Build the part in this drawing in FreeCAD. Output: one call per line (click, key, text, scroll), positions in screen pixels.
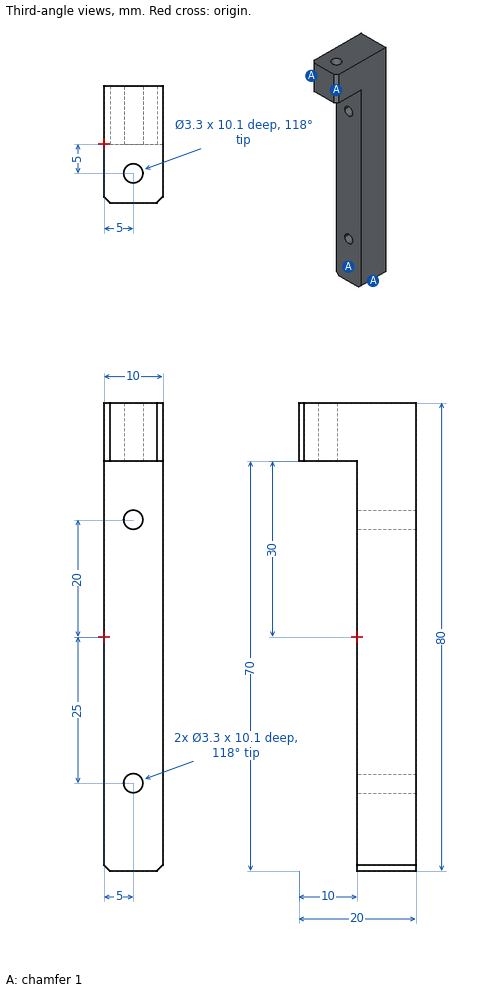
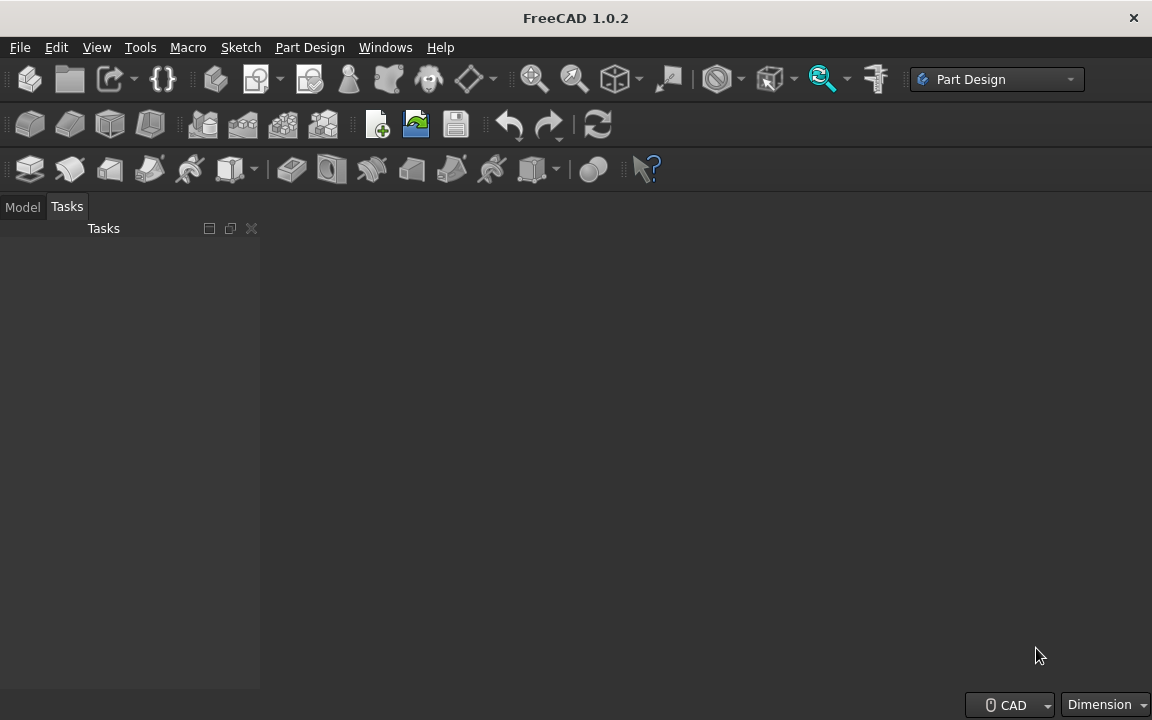
key(ctrl+n)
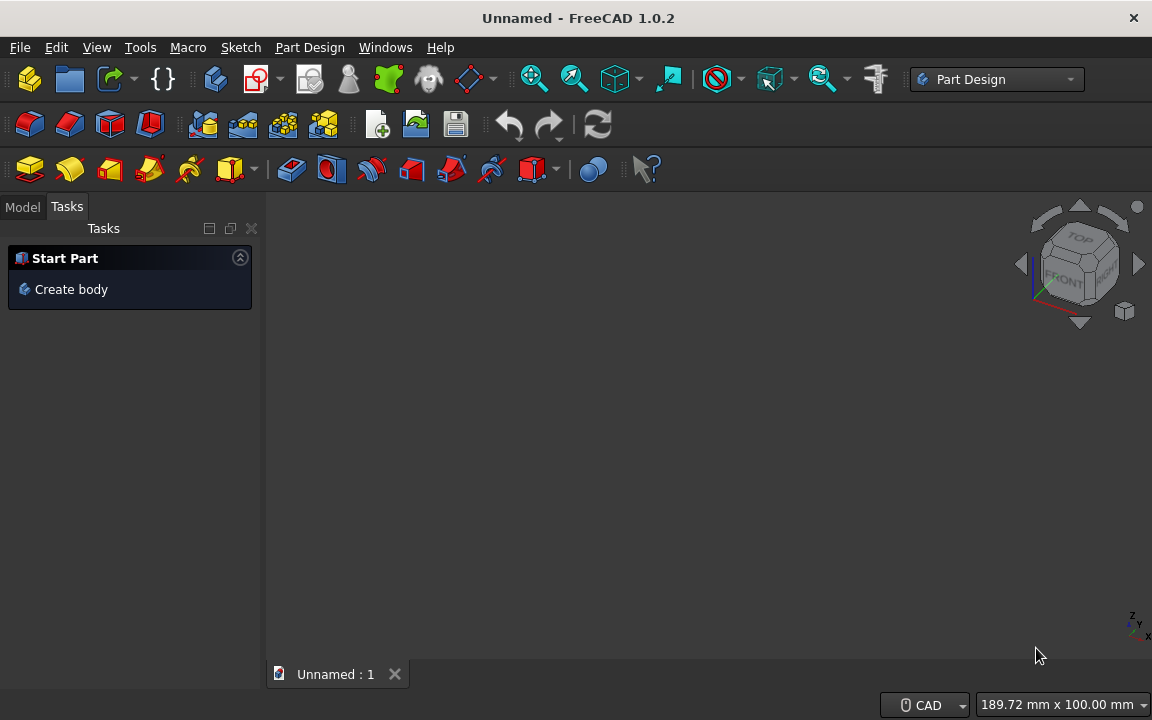
click(256, 80)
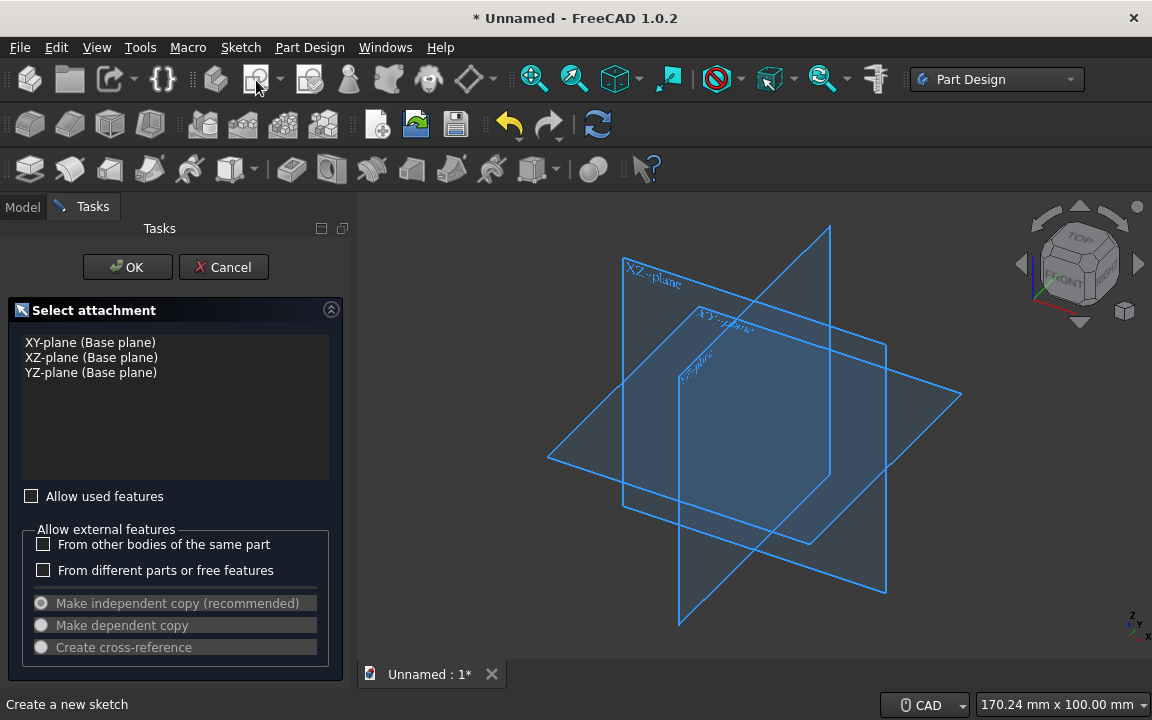
click(82, 372)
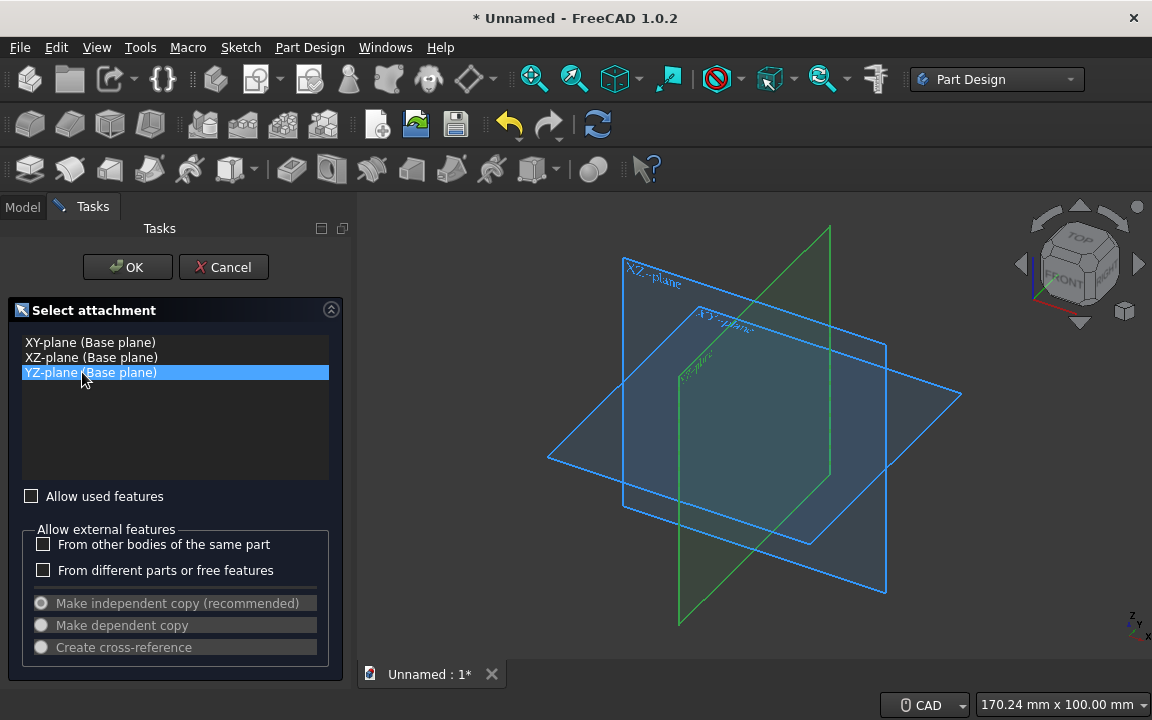
click(128, 267)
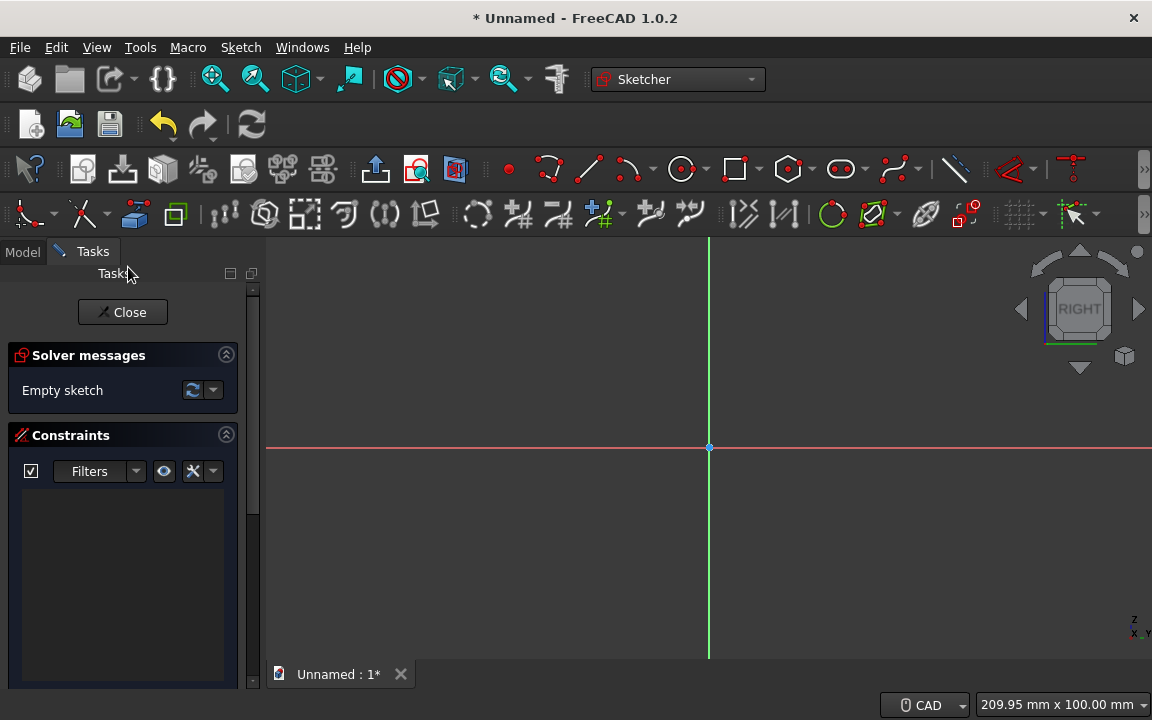
scroll(331, 448, down, 1)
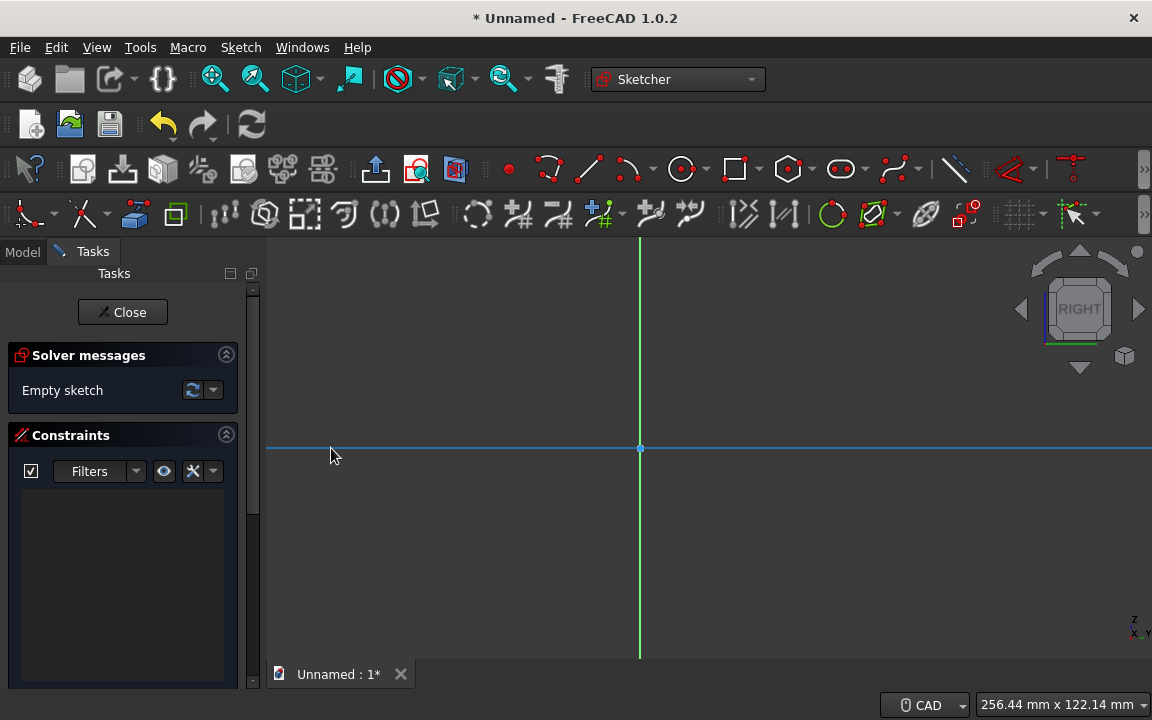
key(g)
key(v)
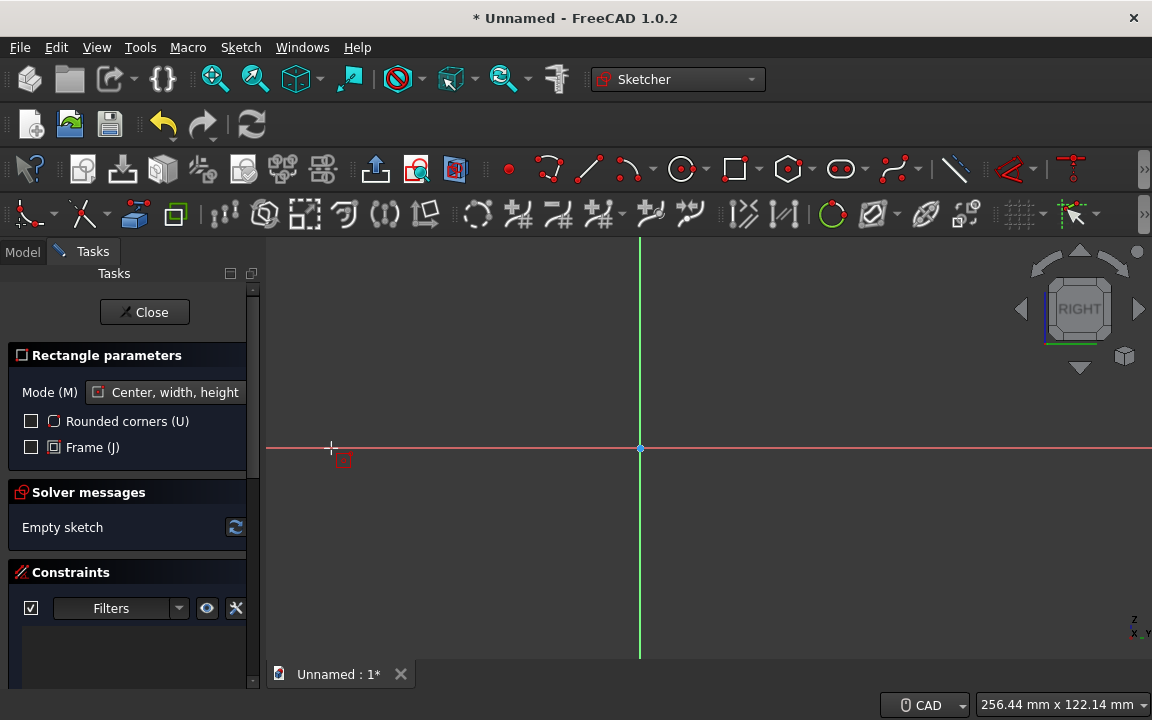
click(640, 448)
move(675, 310)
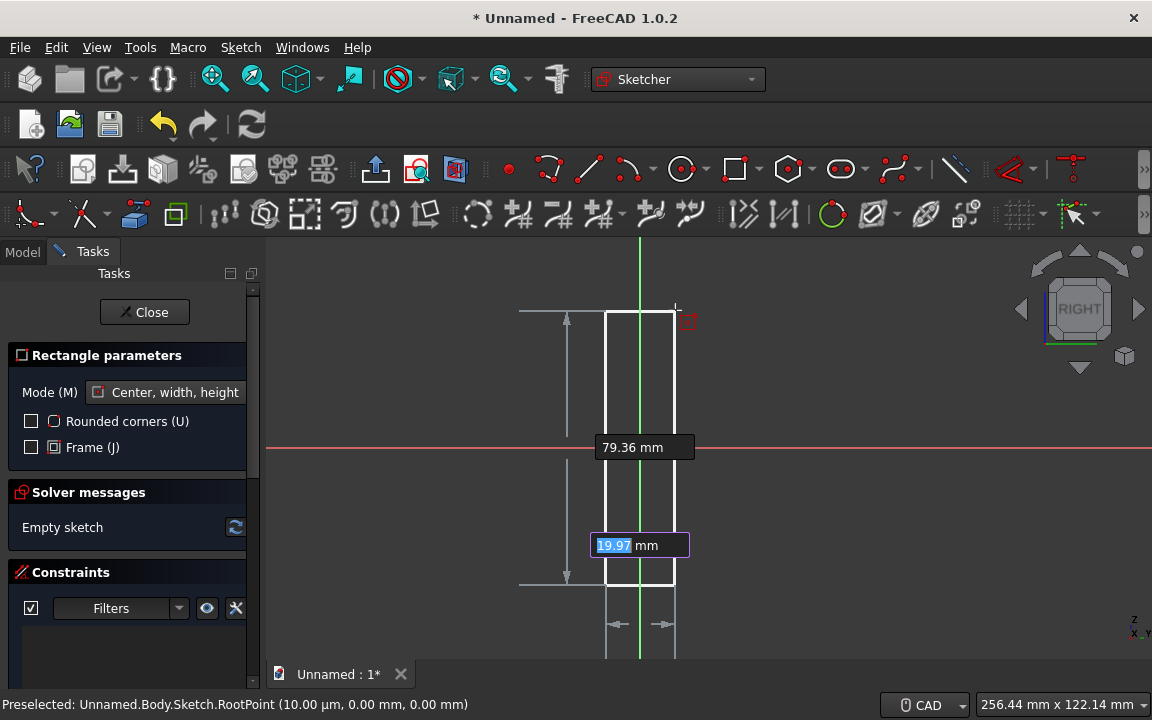
text(20)
key(Tab)
text(80)
key(Return)
key(Escape)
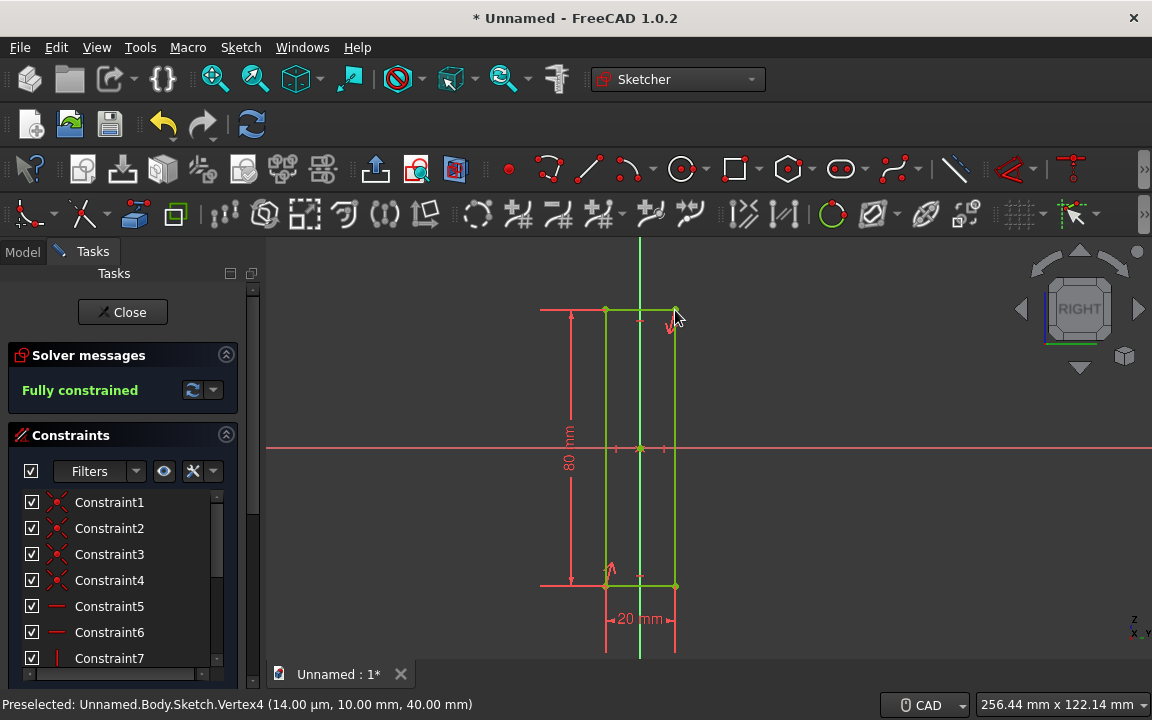
click(123, 312)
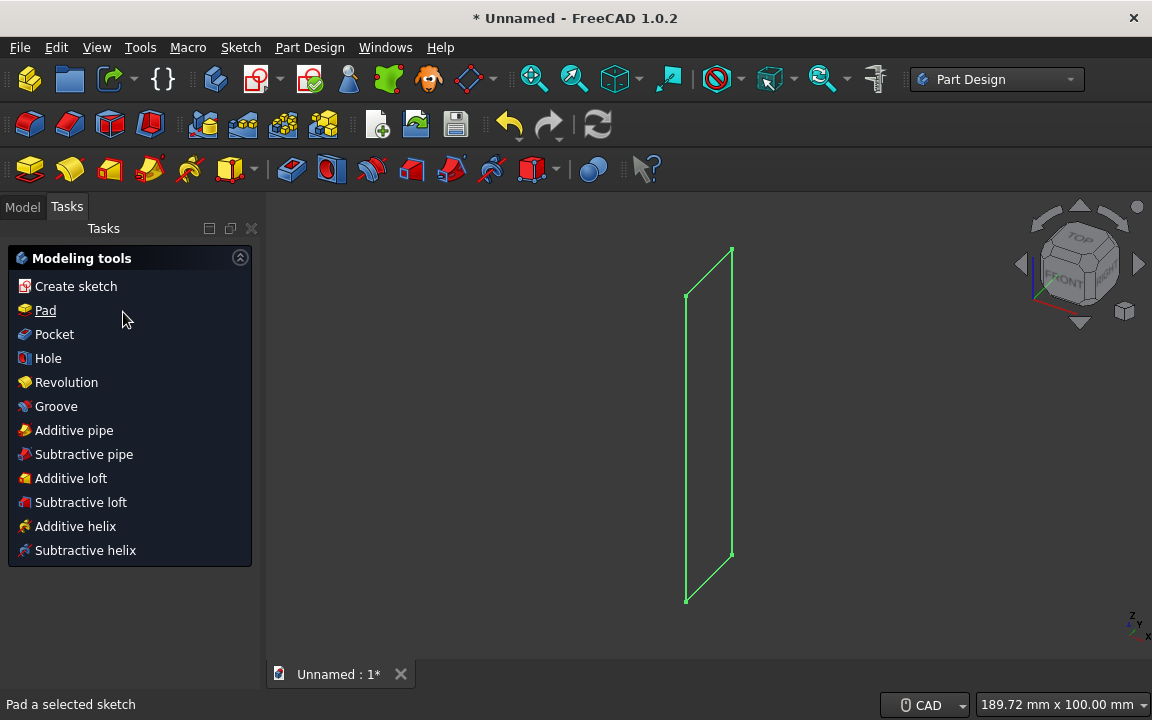
click(30, 170)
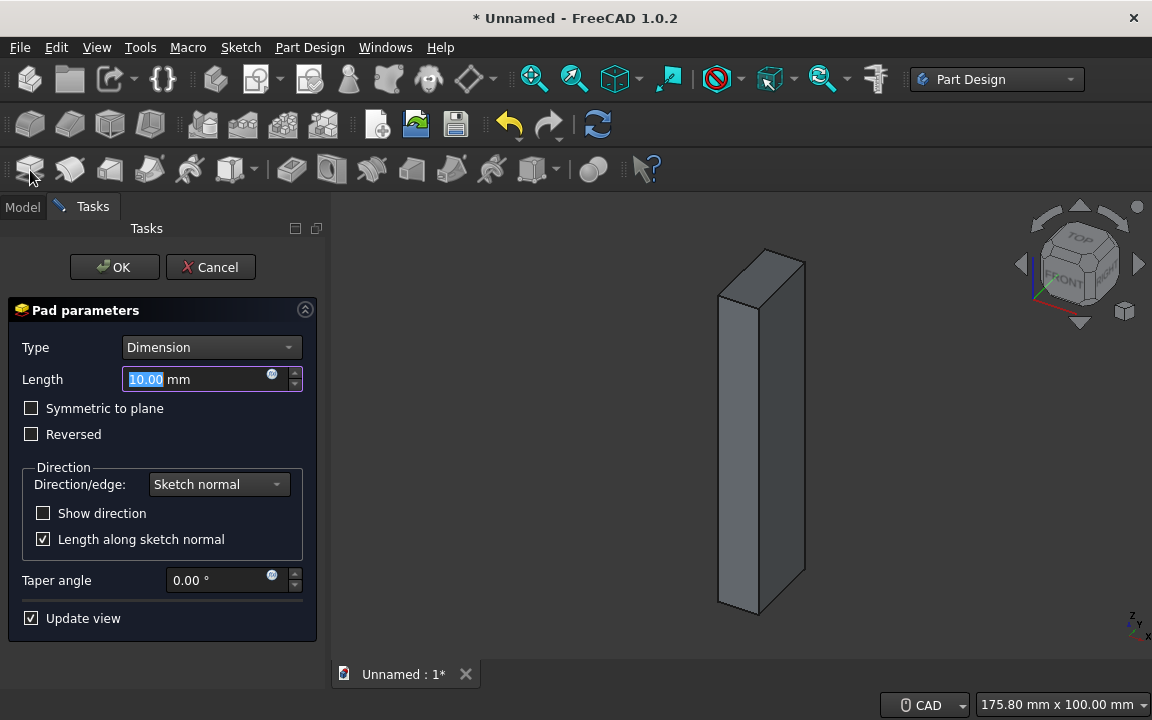
text(10)
key(Tab)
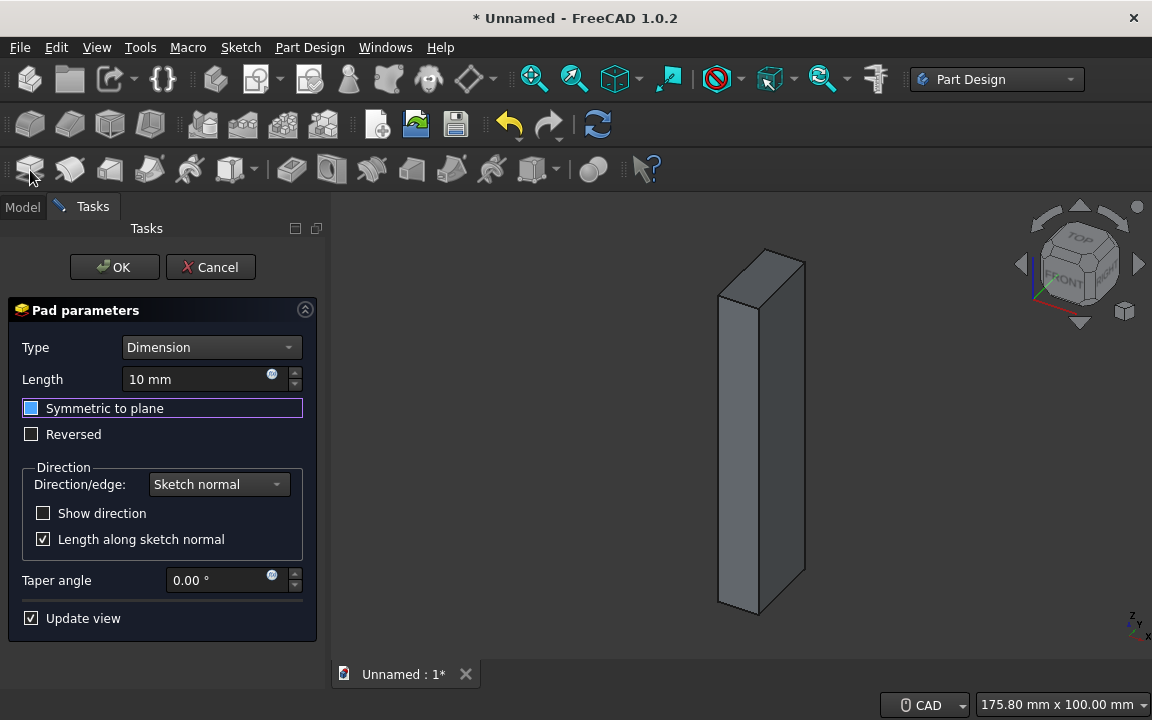
click(115, 267)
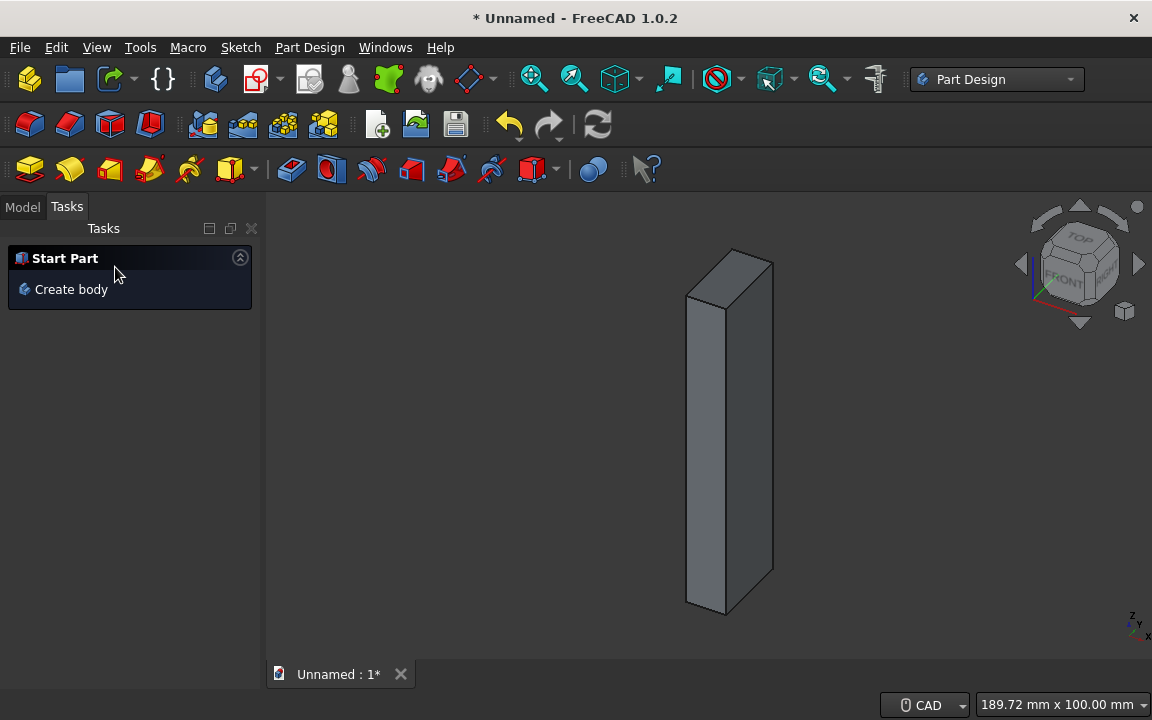
click(256, 80)